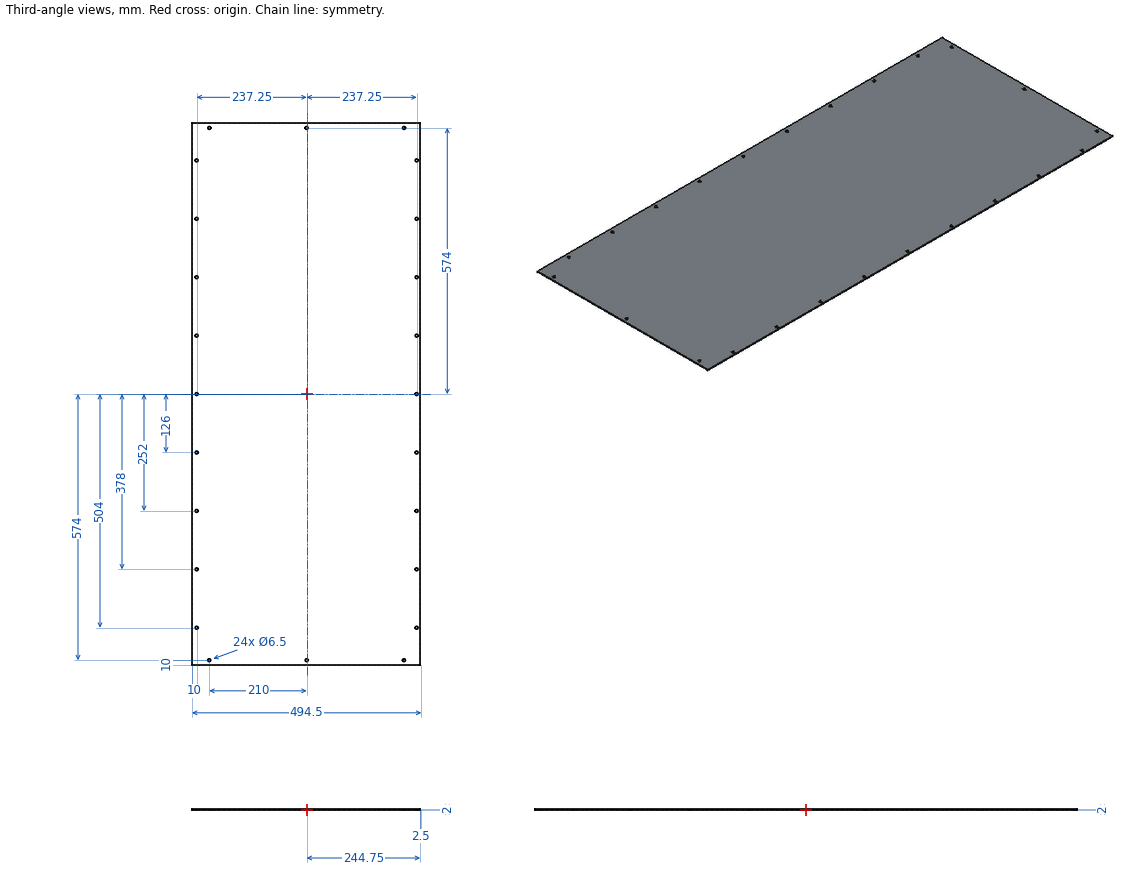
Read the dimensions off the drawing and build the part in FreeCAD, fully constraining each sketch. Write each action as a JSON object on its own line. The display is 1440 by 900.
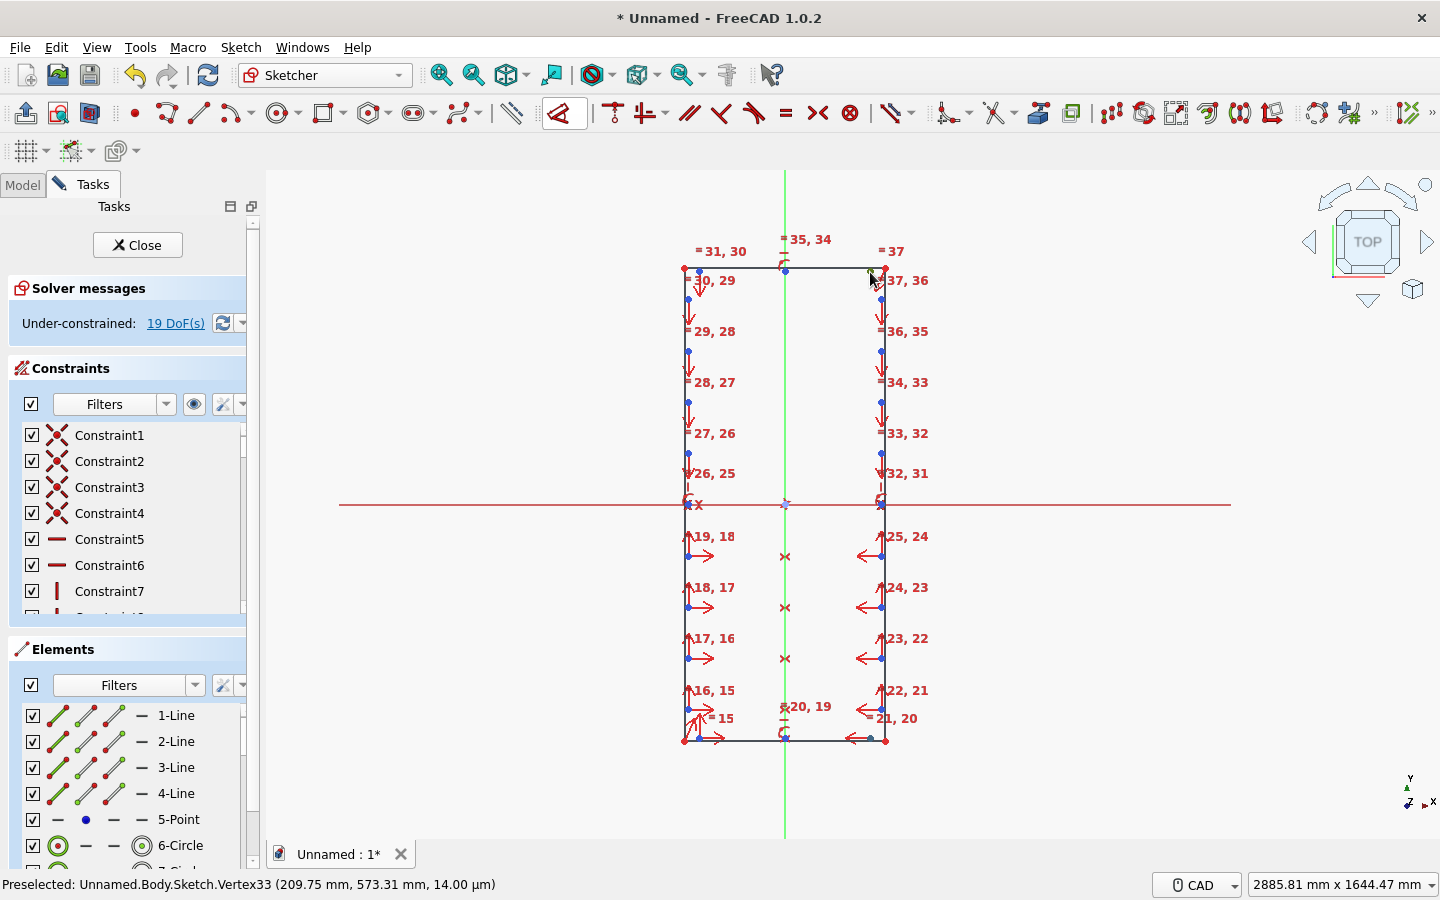
{"action": "left_click", "coordinate": [364, 505]}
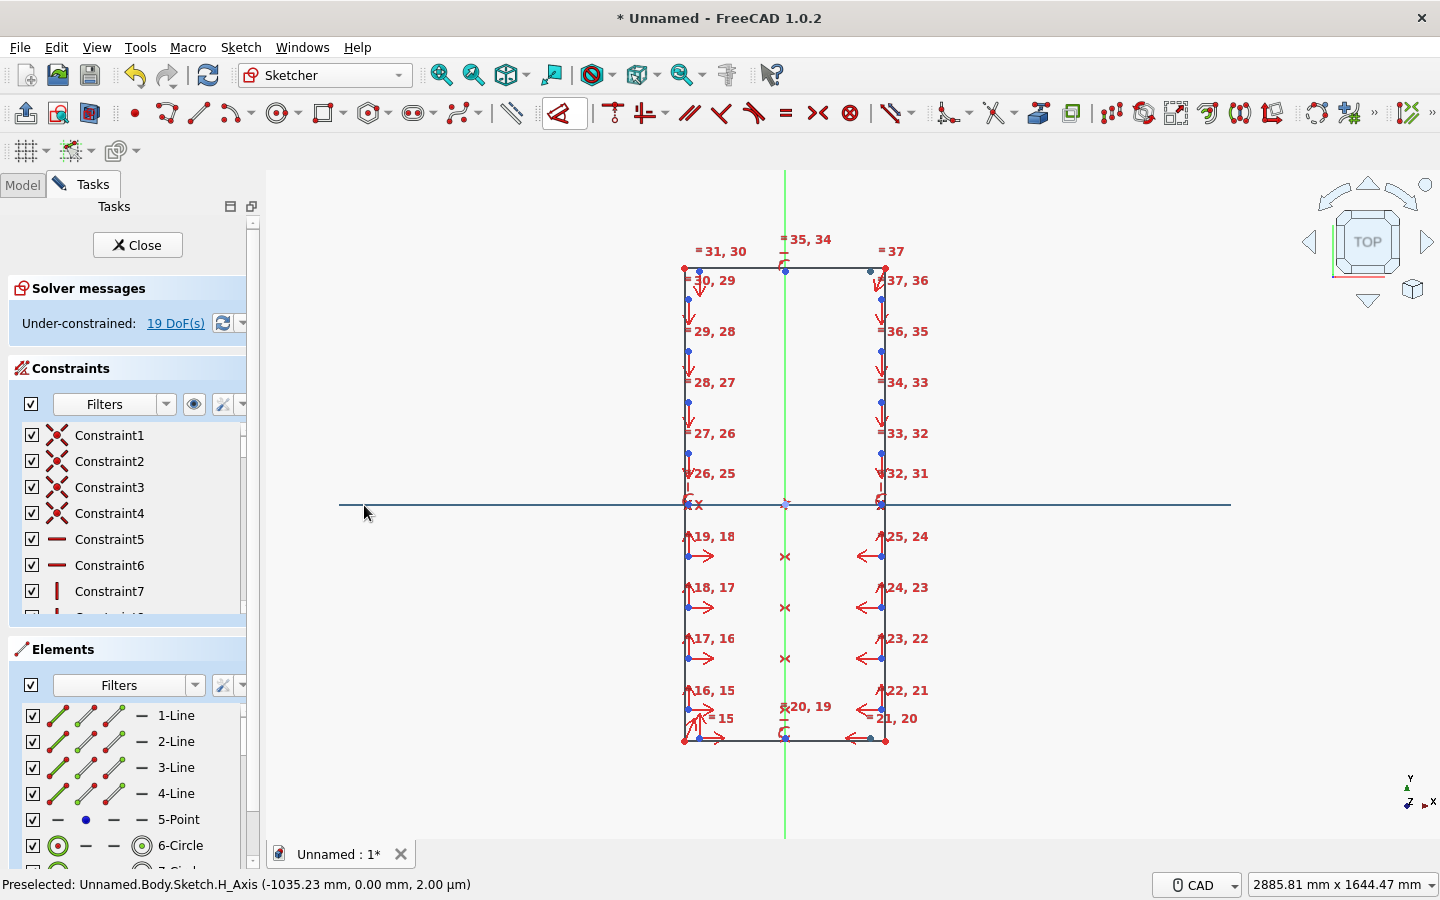
{"action": "left_click", "coordinate": [818, 114]}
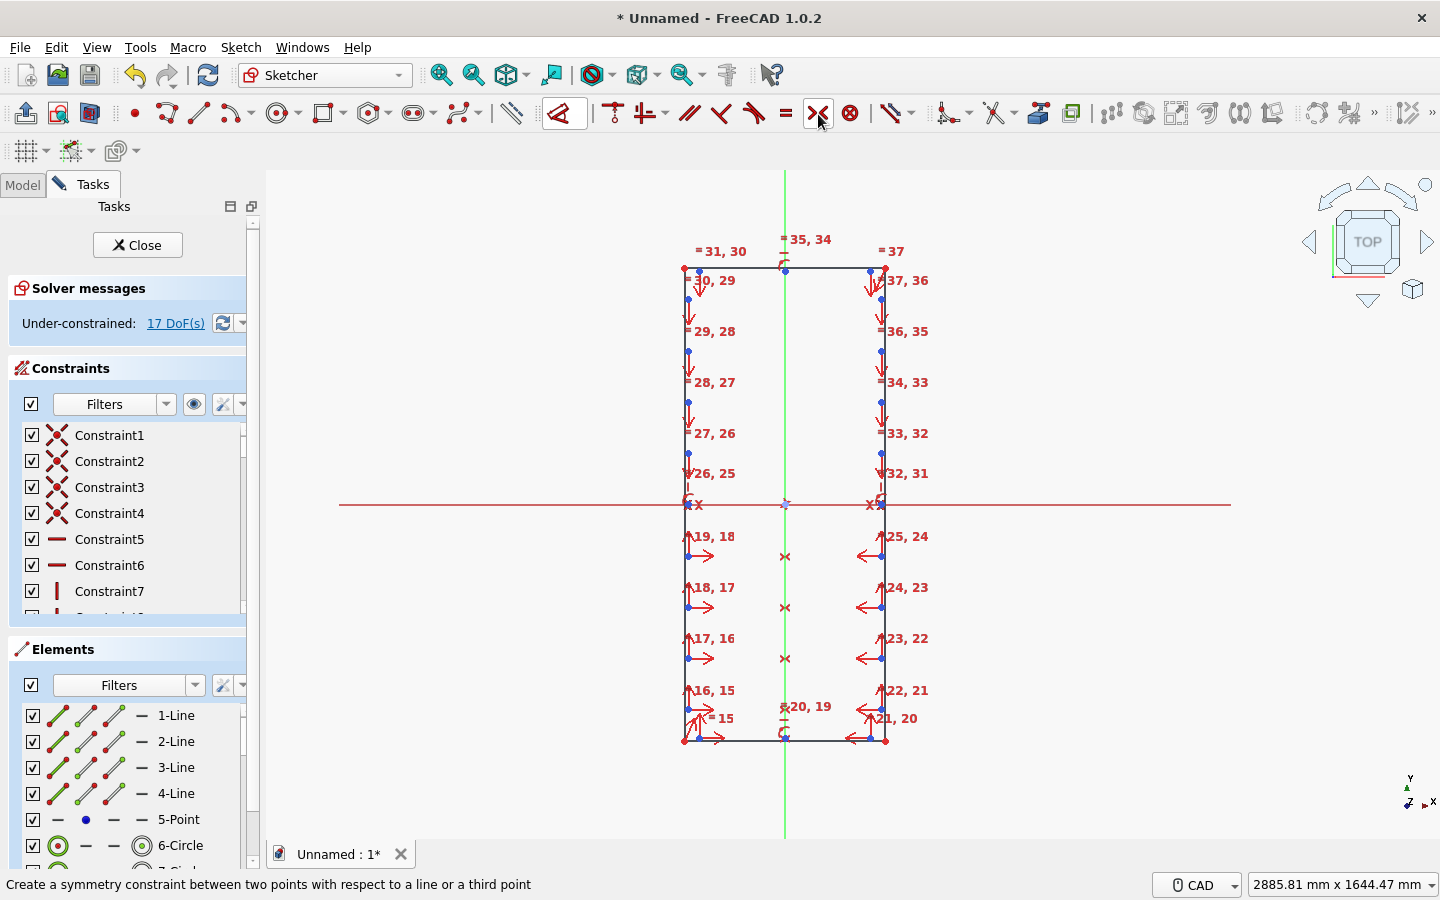
{"action": "scroll", "coordinate": [700, 737], "scroll_direction": "up", "scroll_amount": 14}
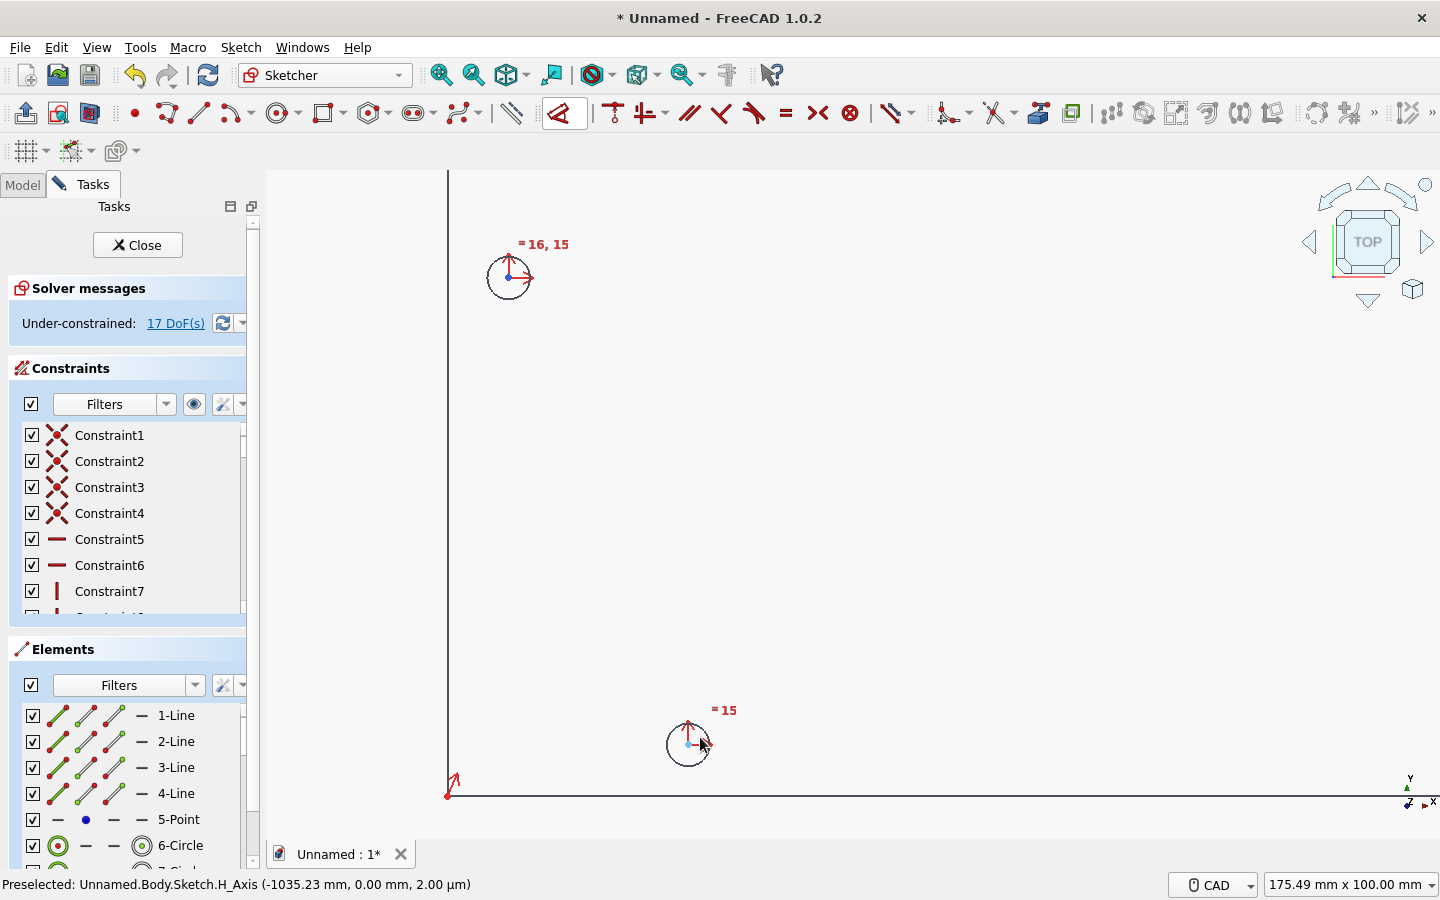
{"action": "left_click", "coordinate": [689, 724]}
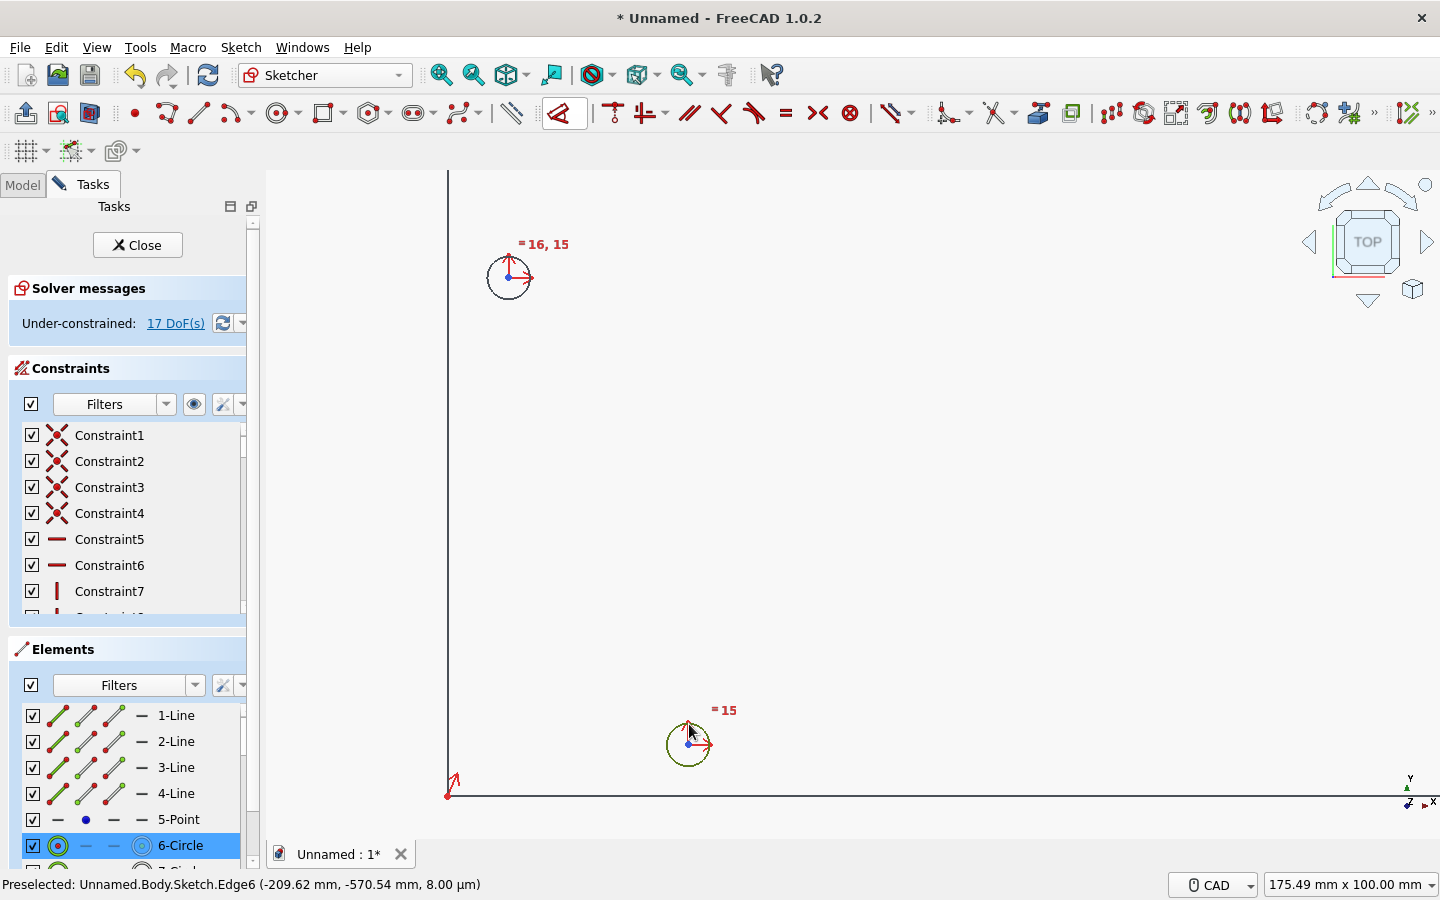
{"action": "key", "text": "k o"}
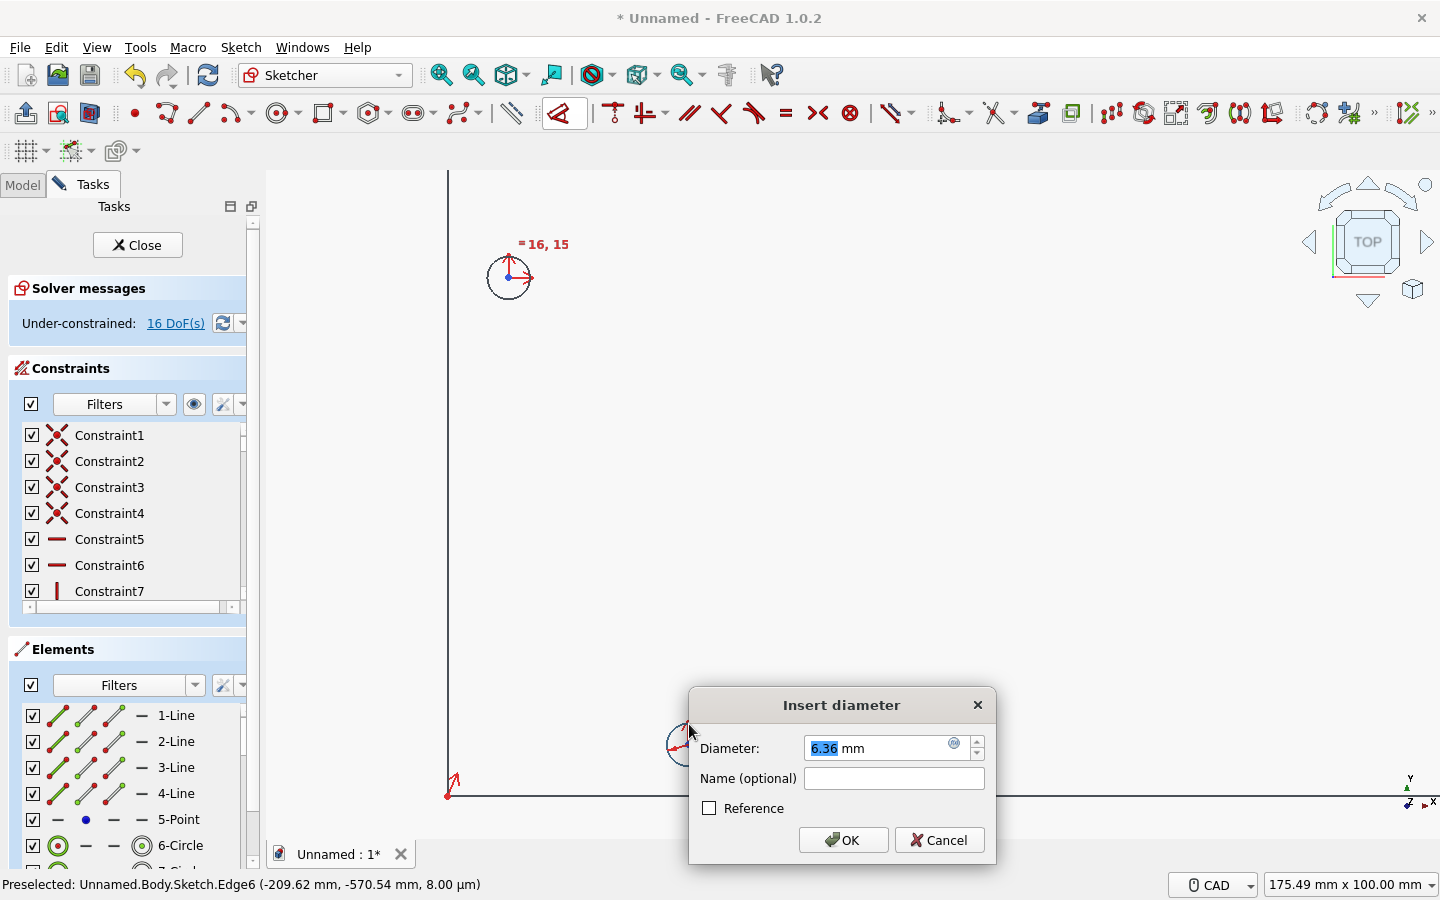
{"action": "type", "text": "6.5"}
{"action": "key", "text": "Return"}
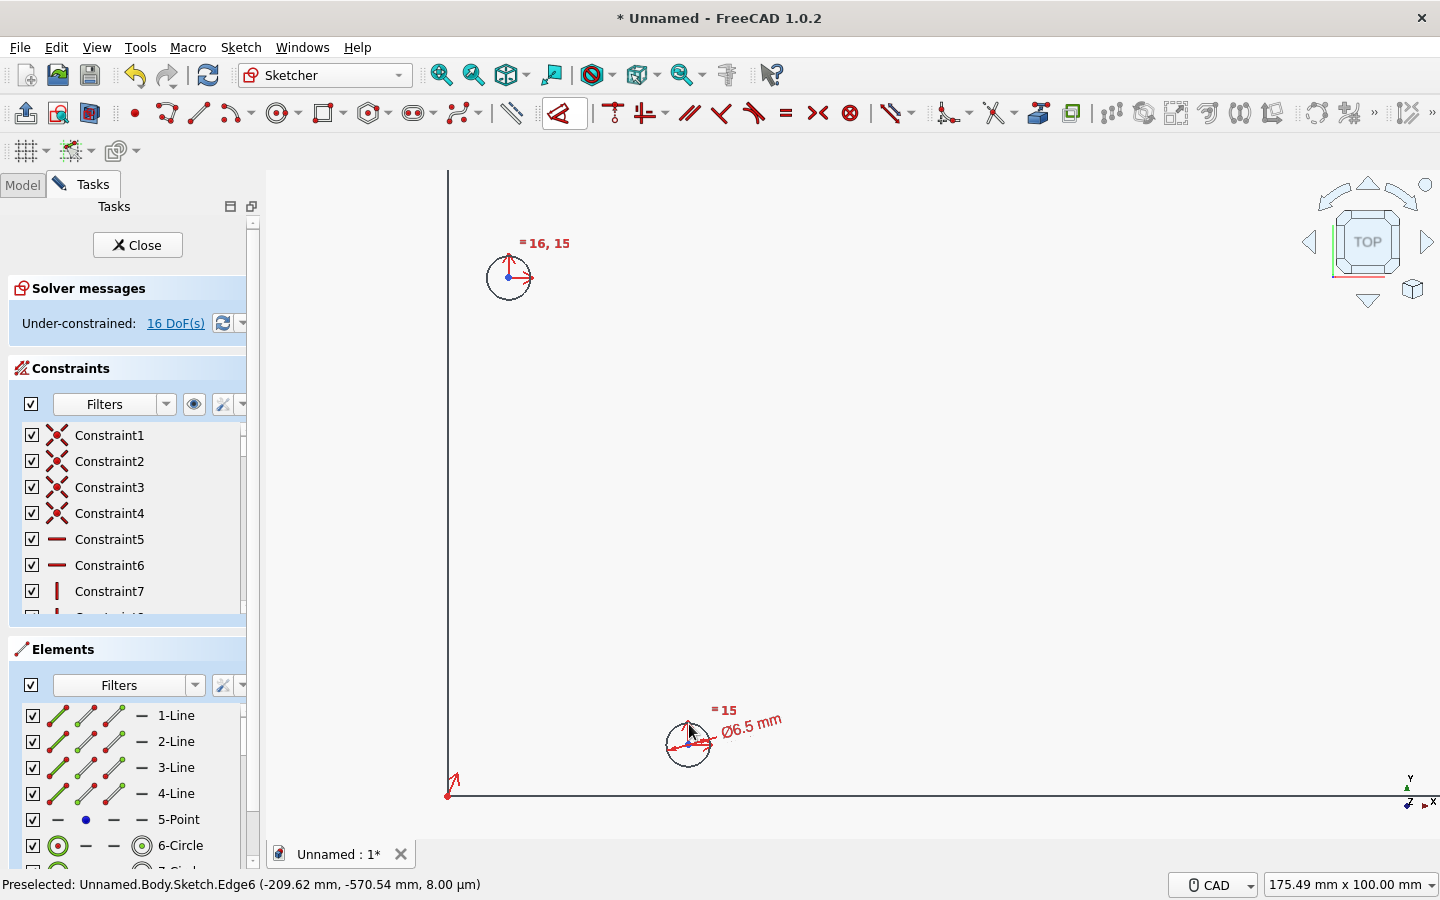
{"action": "scroll", "coordinate": [700, 737], "scroll_direction": "down", "scroll_amount": 14}